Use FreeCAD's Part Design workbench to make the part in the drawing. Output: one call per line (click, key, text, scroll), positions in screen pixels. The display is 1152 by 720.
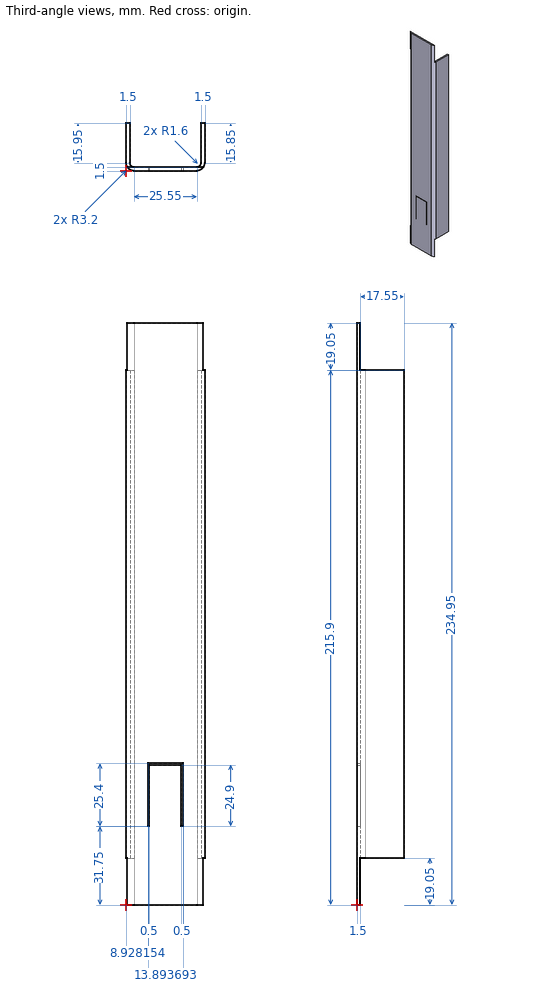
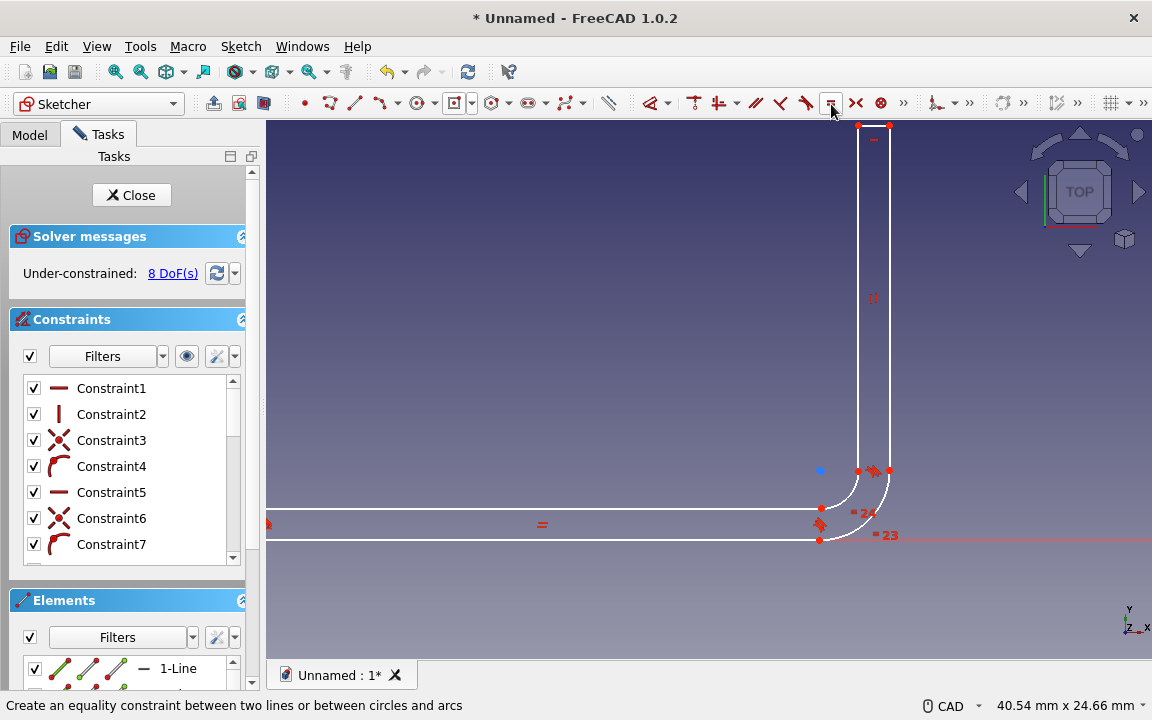
click(650, 104)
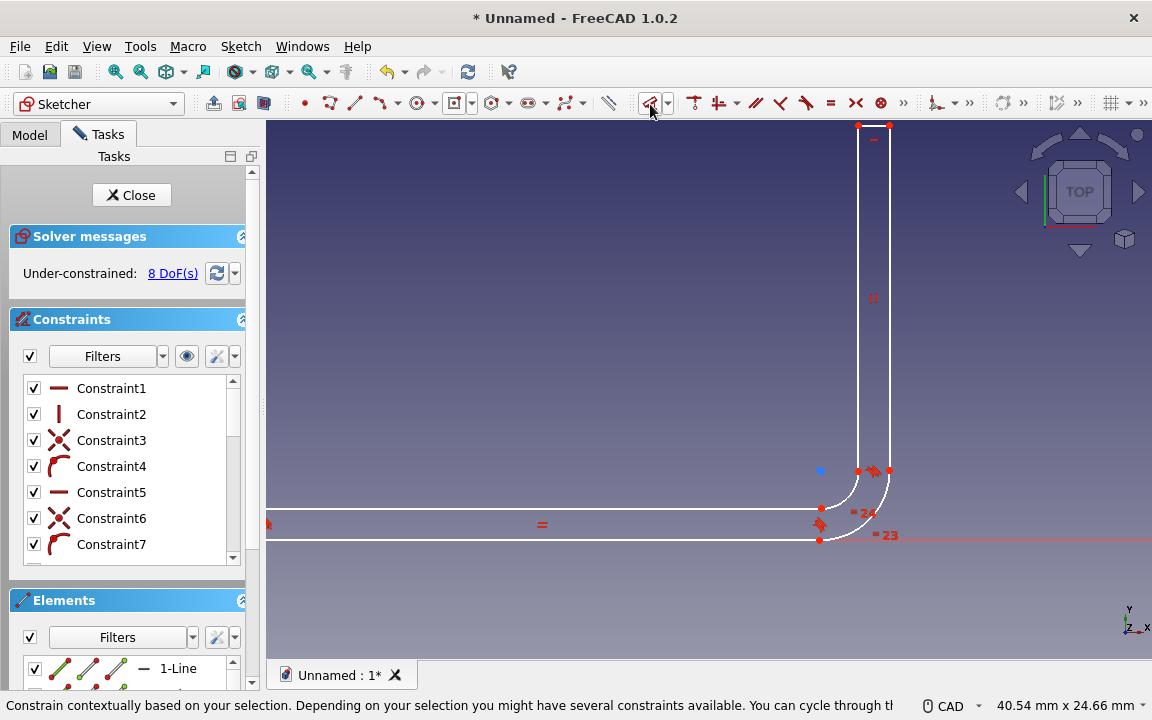
scroll(838, 506, down, 2)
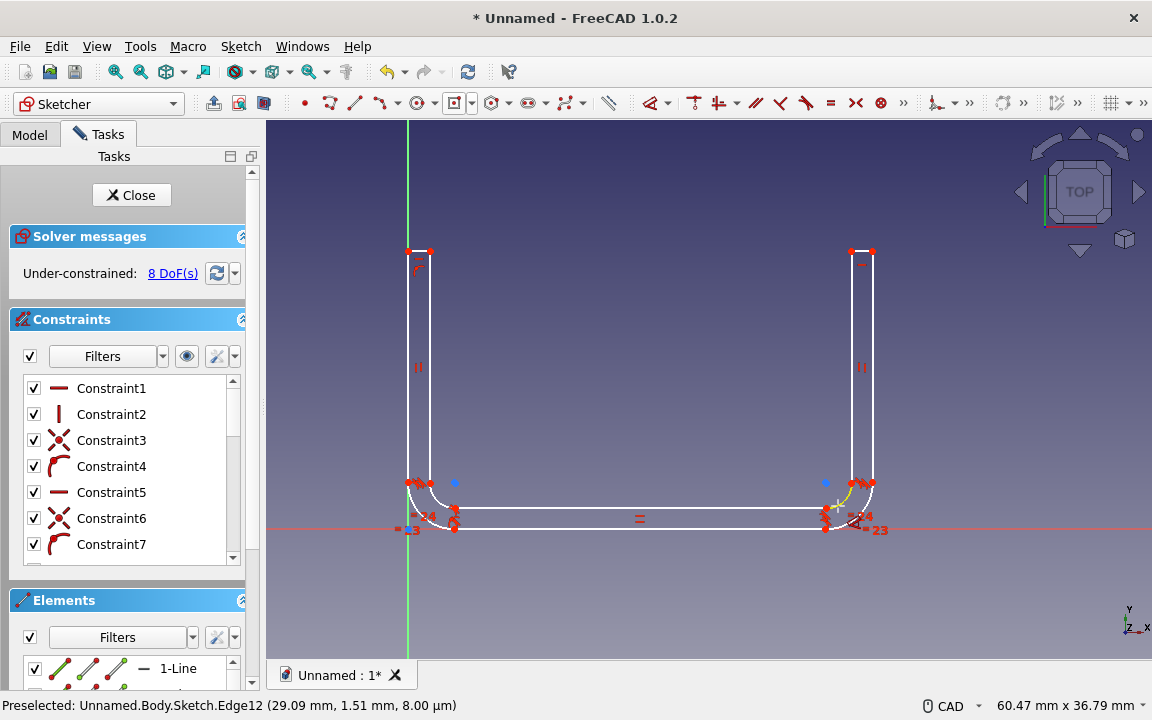
scroll(433, 495, up, 3)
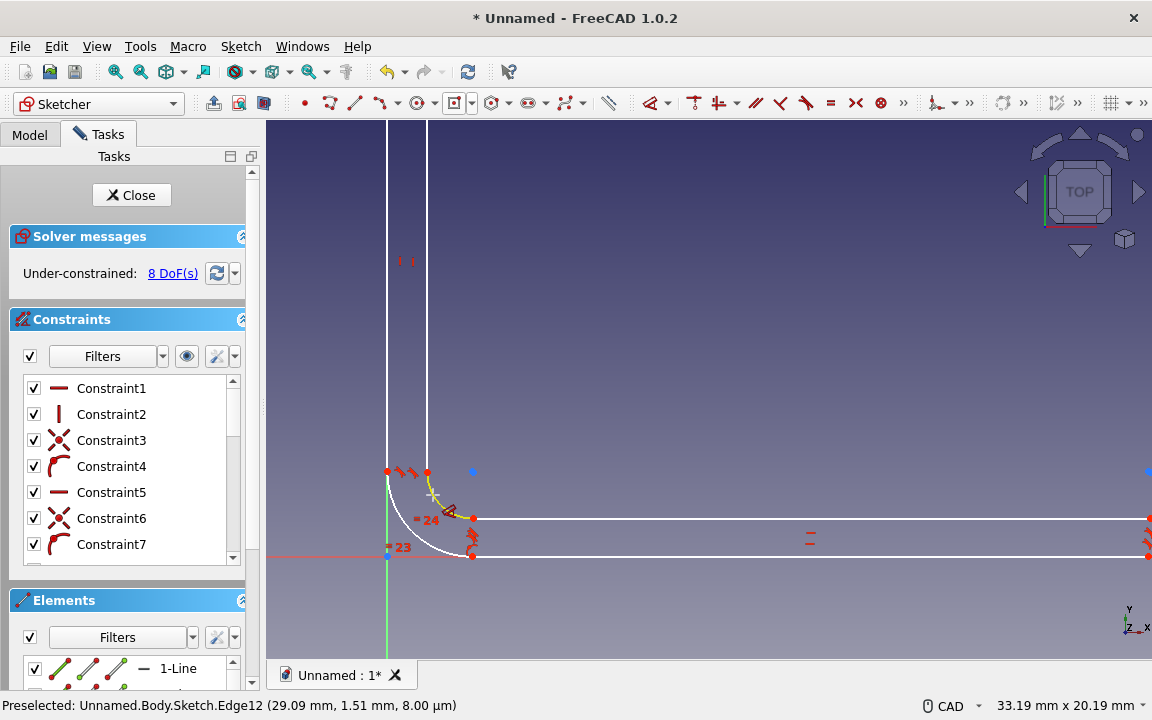
click(432, 494)
click(405, 434)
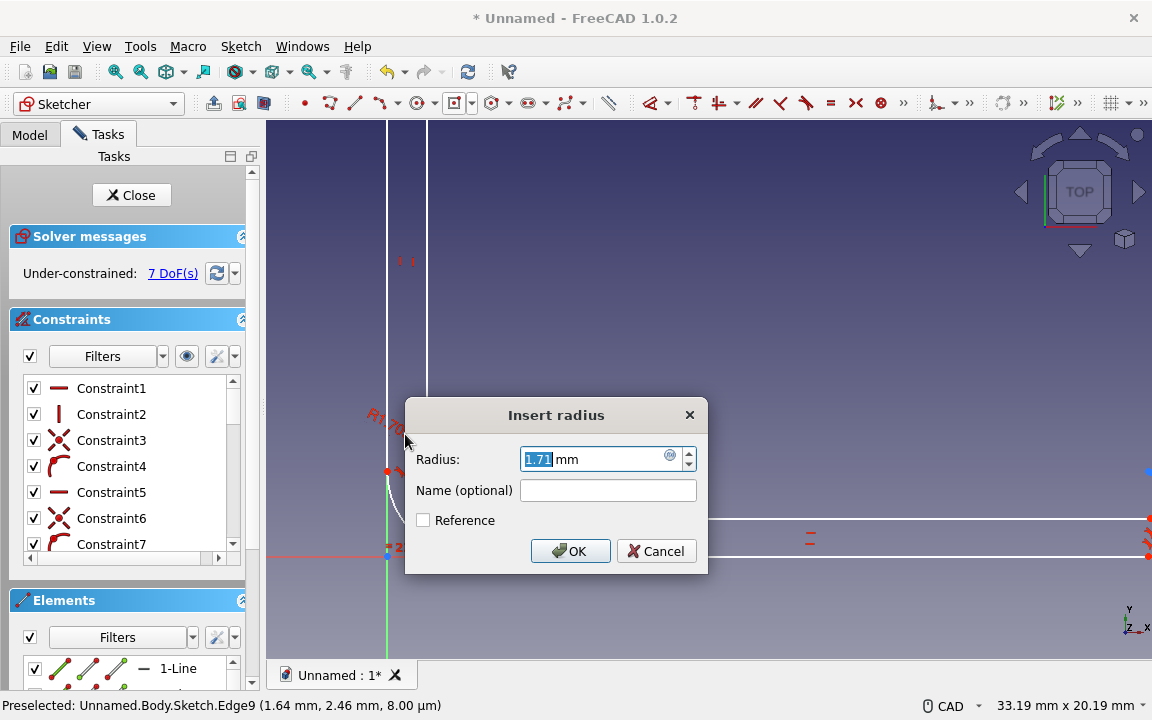
text(1.6)
key(Return)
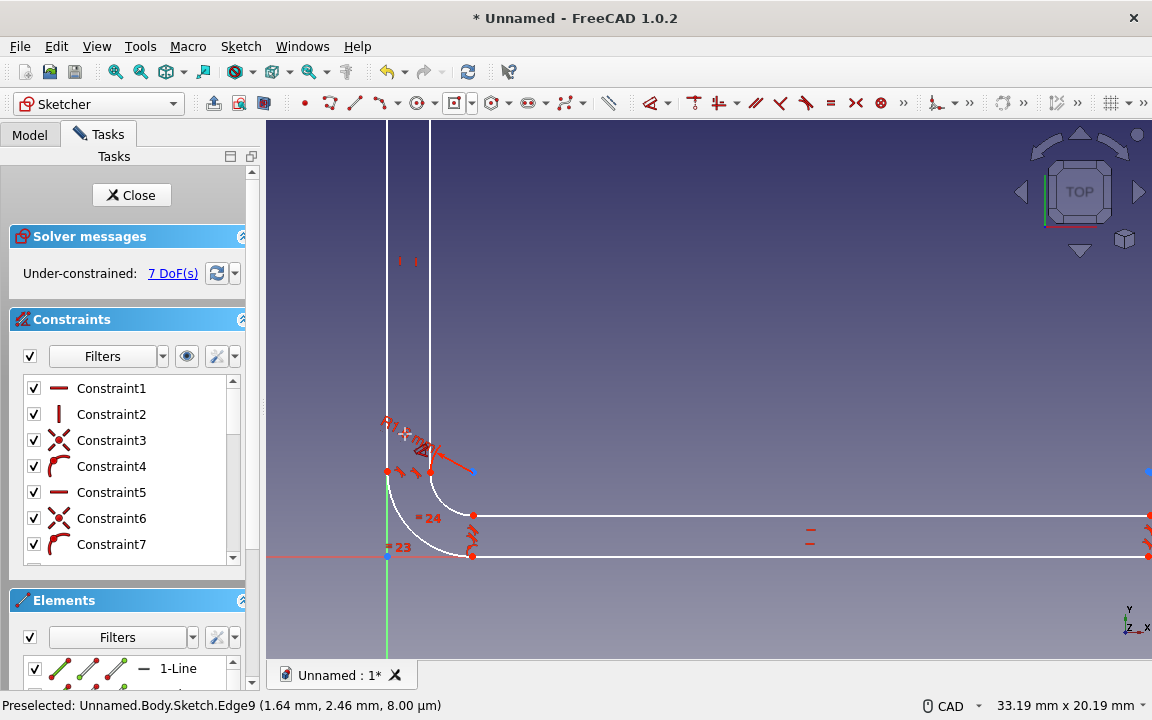
scroll(397, 510, up, 2)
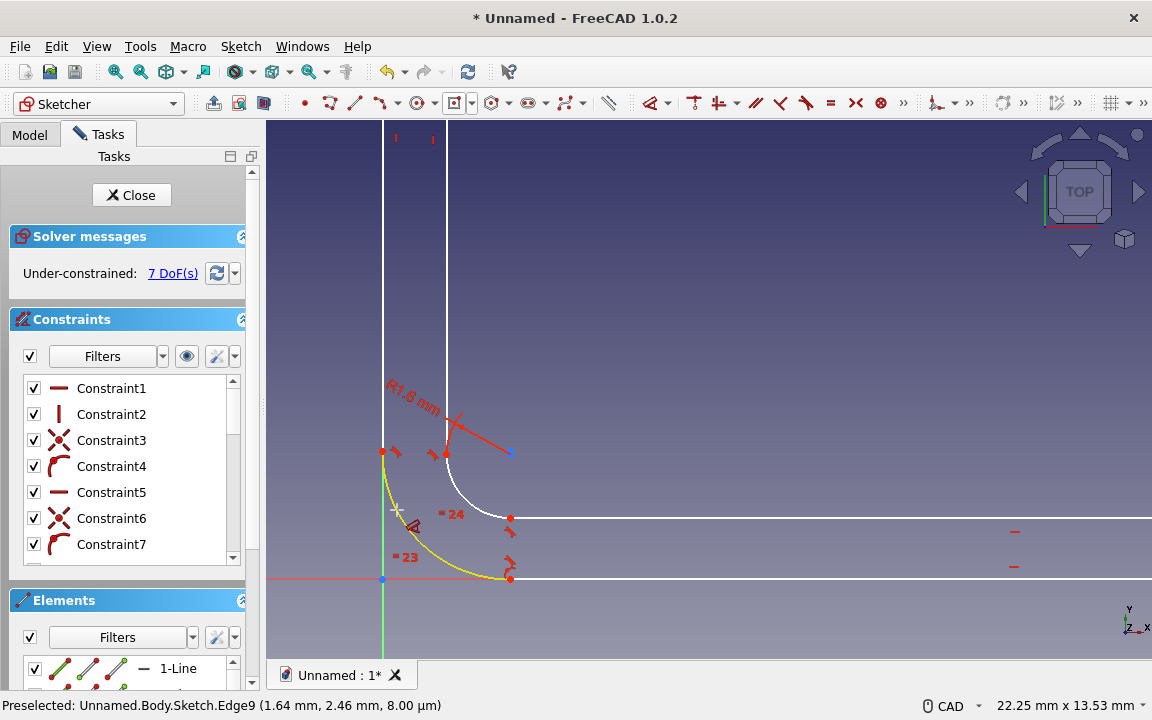
click(396, 510)
click(367, 525)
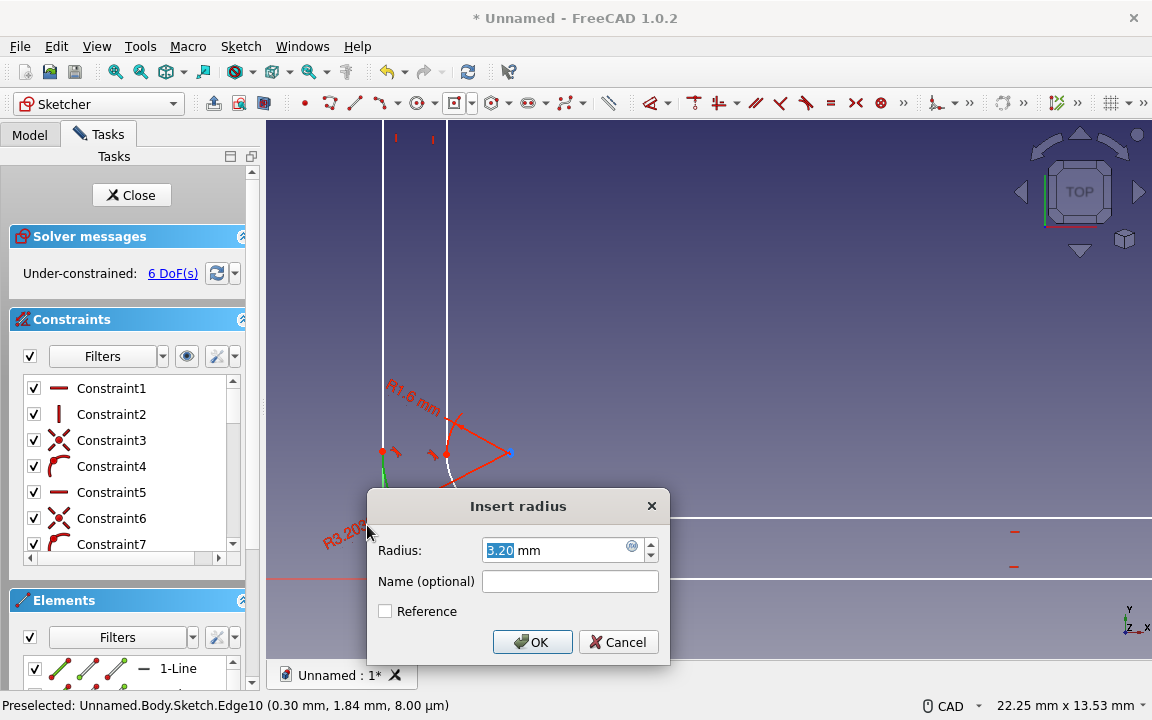
text(3.2)
key(Return)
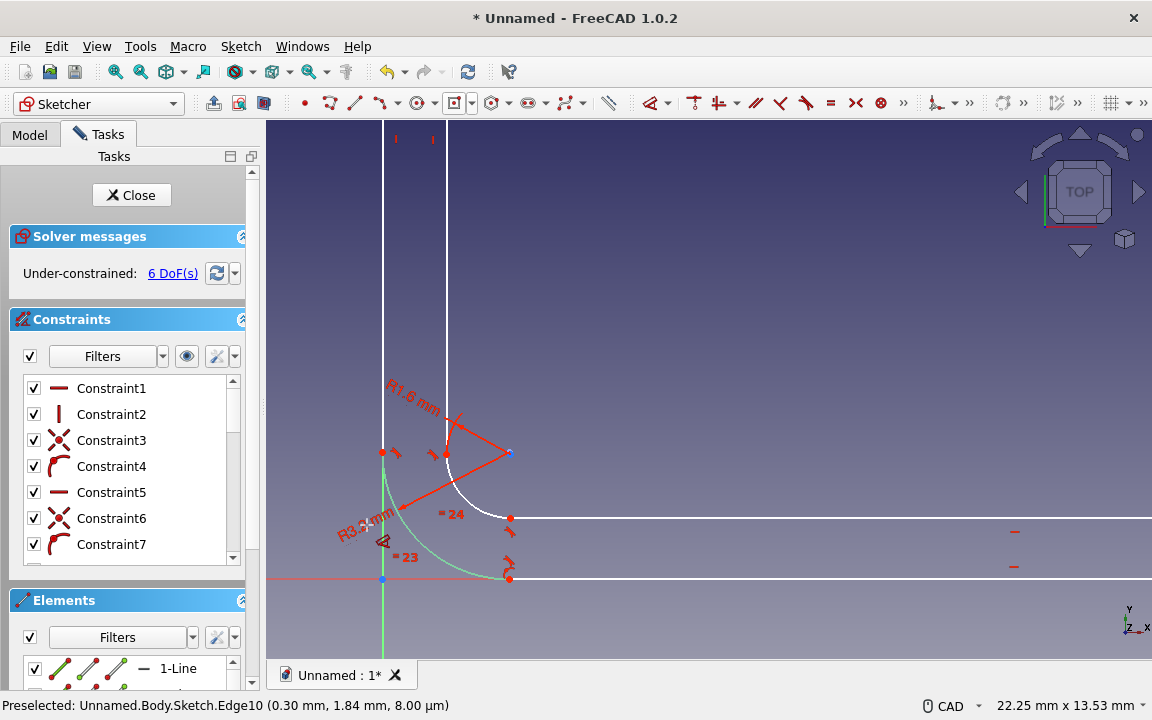
scroll(423, 500, down, 5)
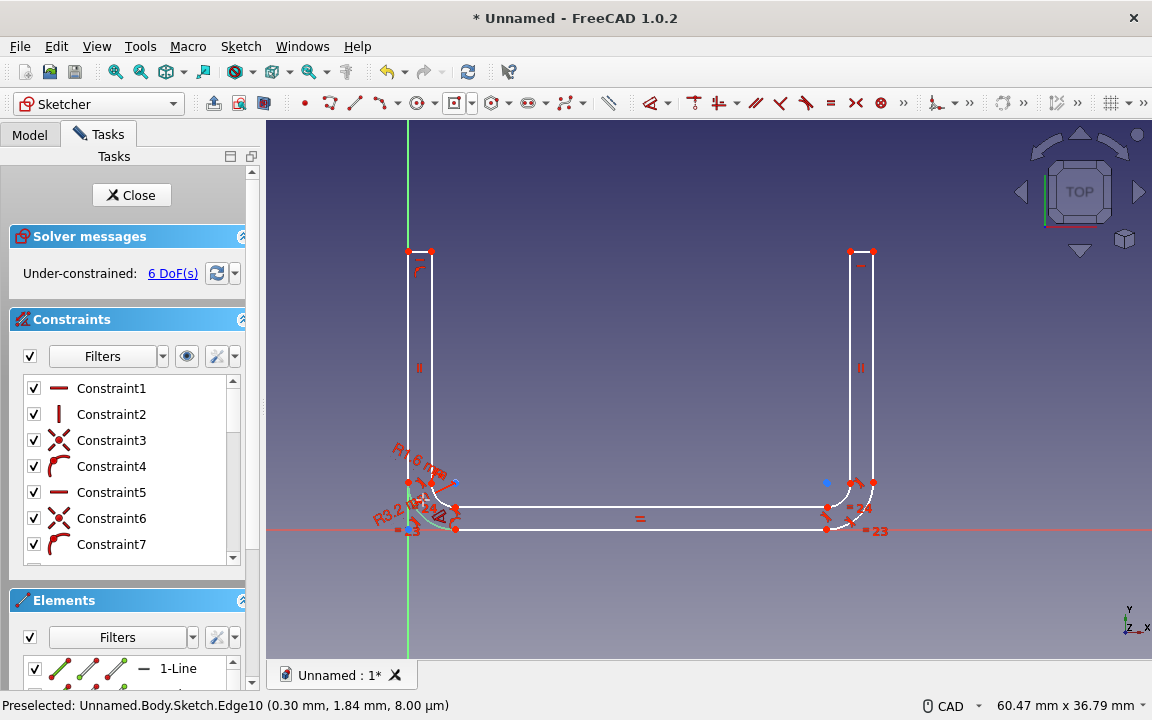
scroll(425, 252, up, 4)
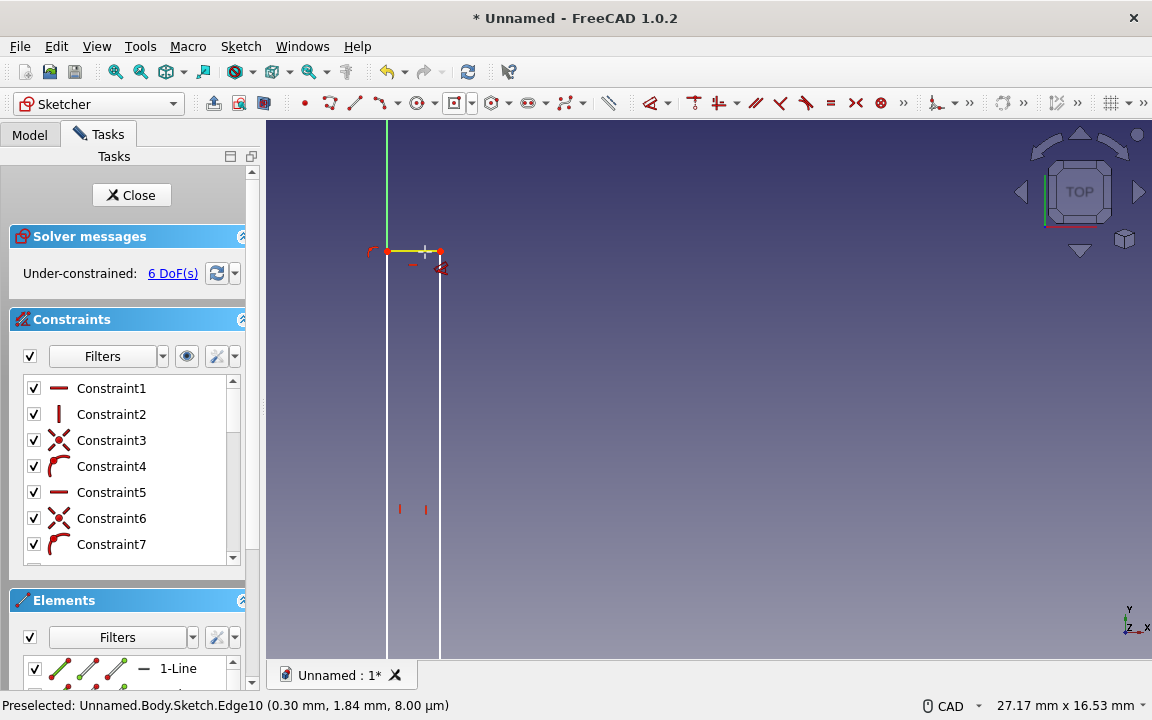
click(424, 251)
click(414, 217)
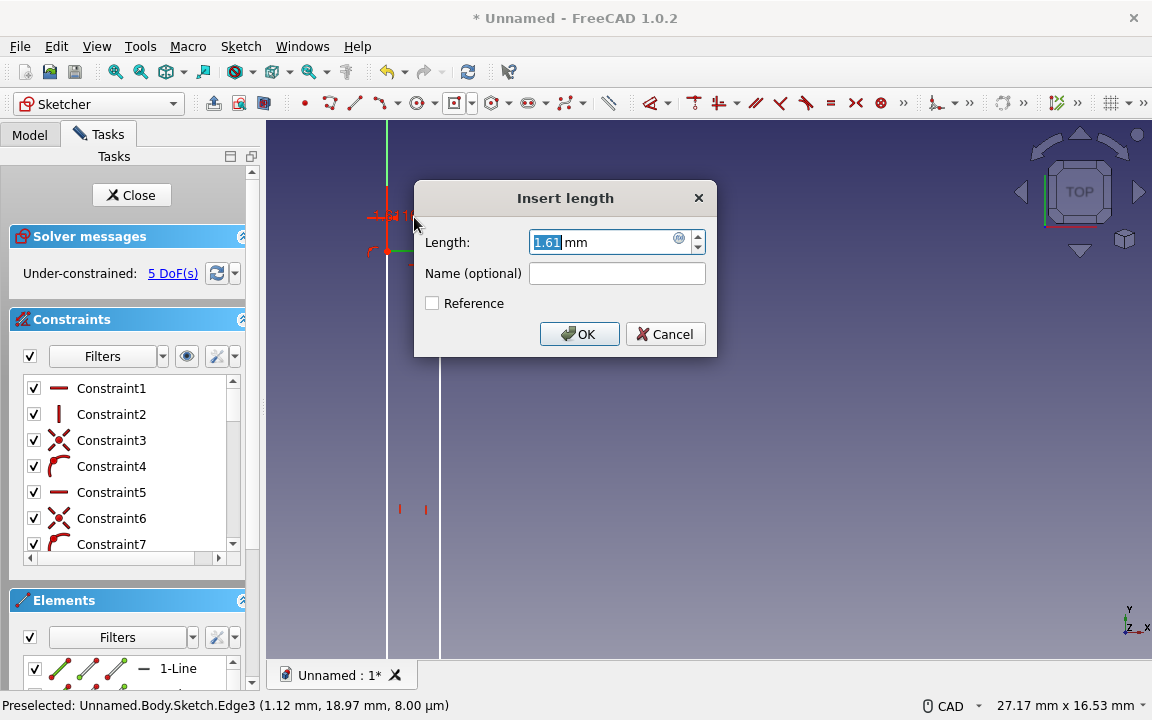
text(1.5)
key(Return)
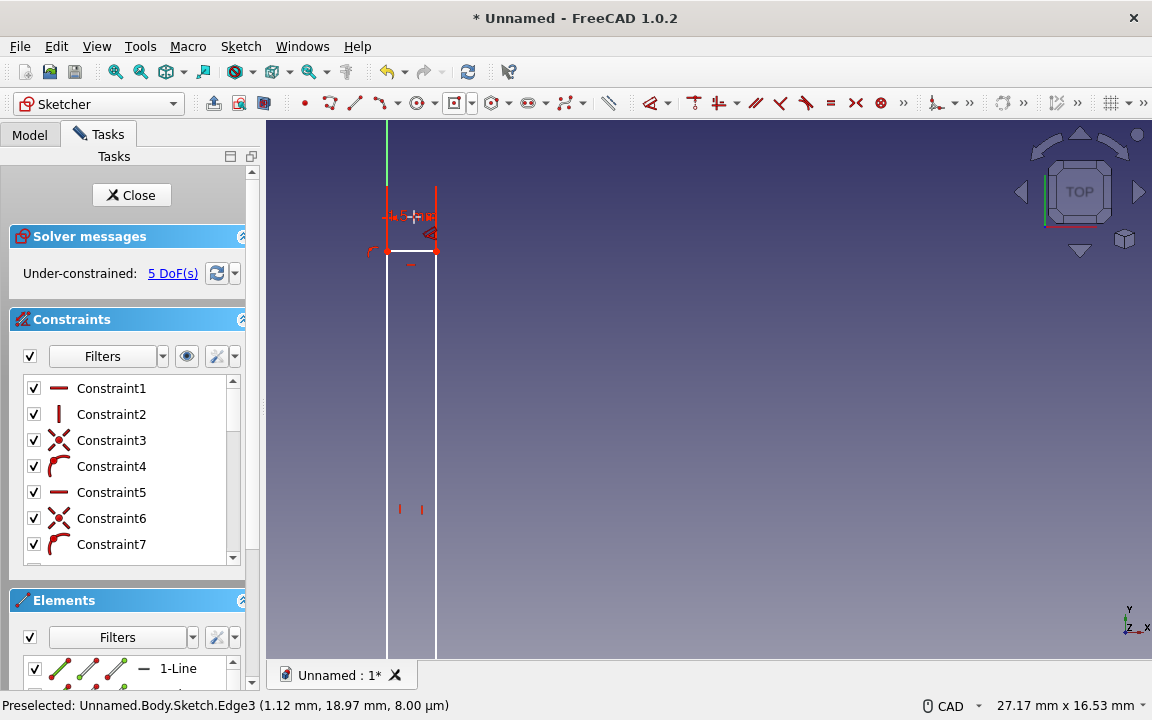
scroll(425, 251, down, 4)